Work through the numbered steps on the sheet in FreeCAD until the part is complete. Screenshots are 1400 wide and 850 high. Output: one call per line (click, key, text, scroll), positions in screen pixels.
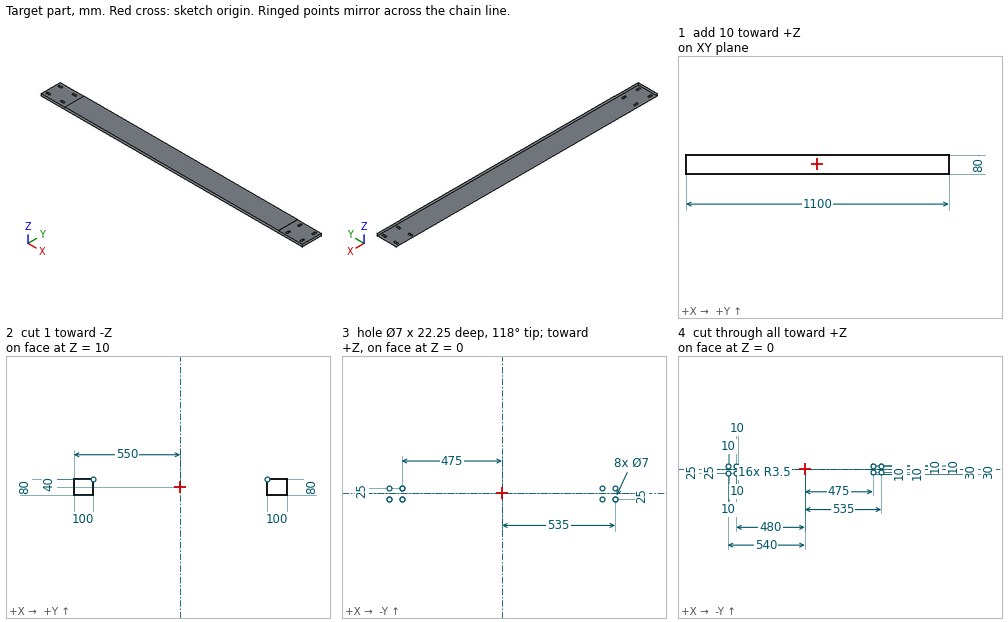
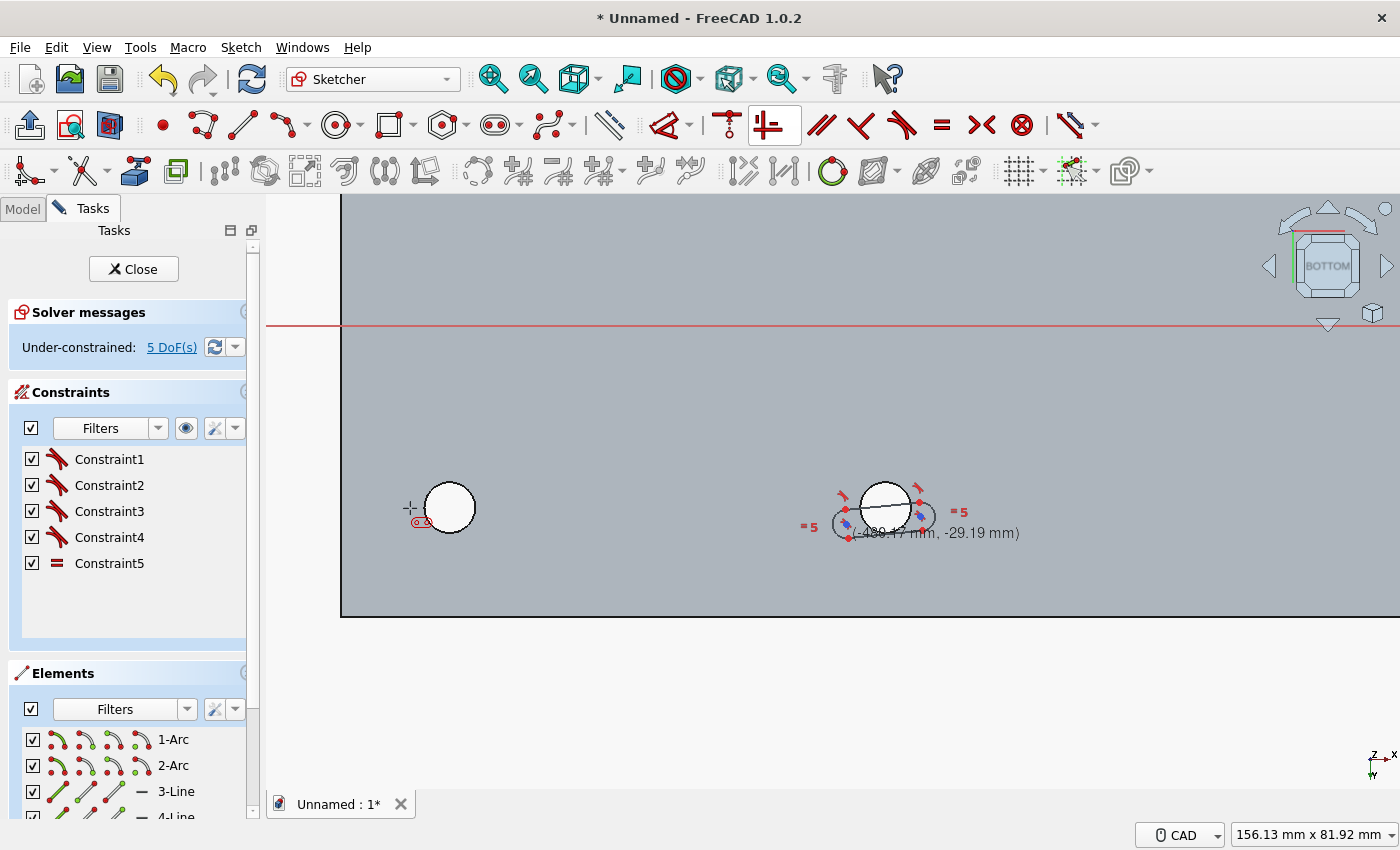
scroll(410, 508, down, 12)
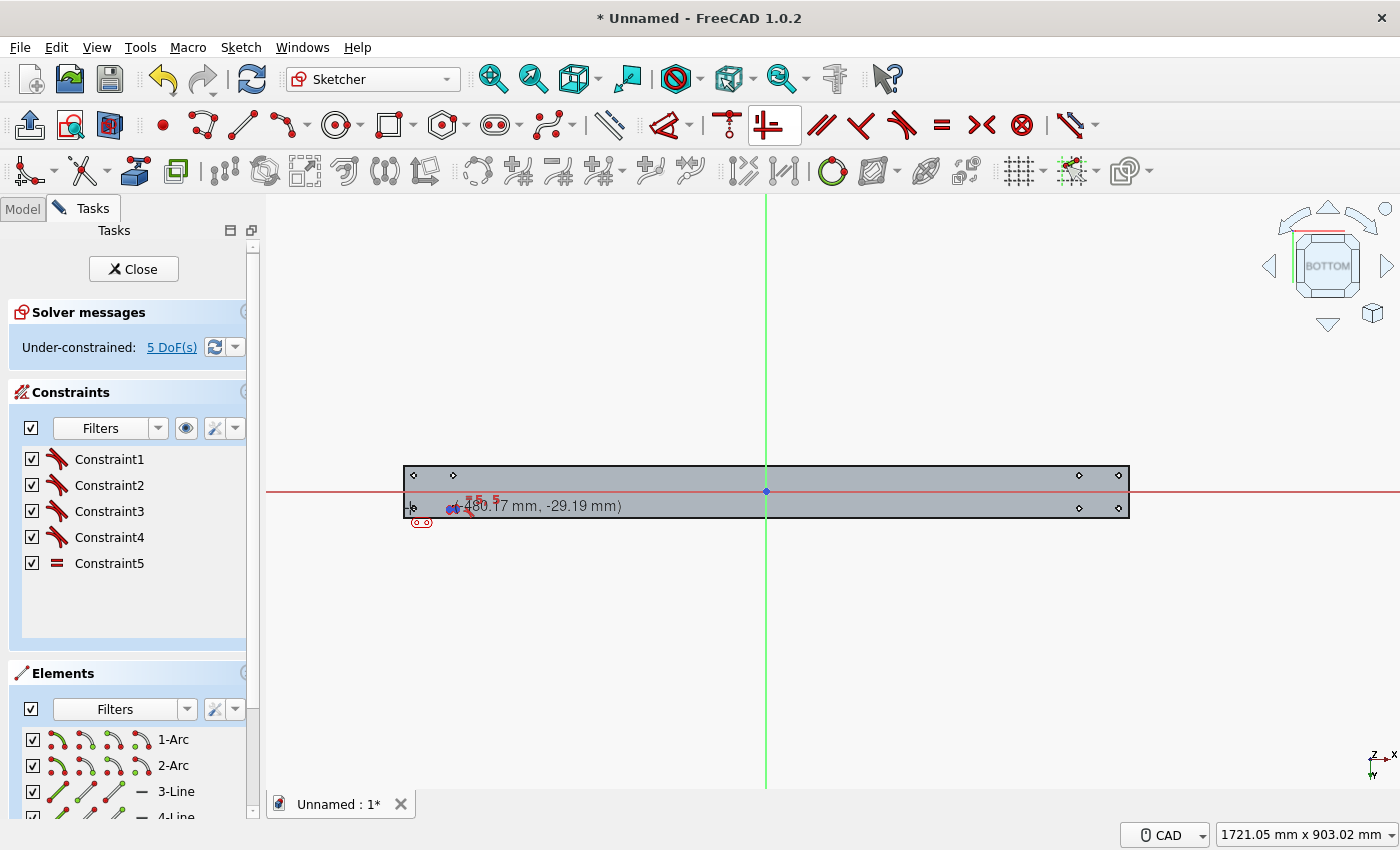
click(410, 508)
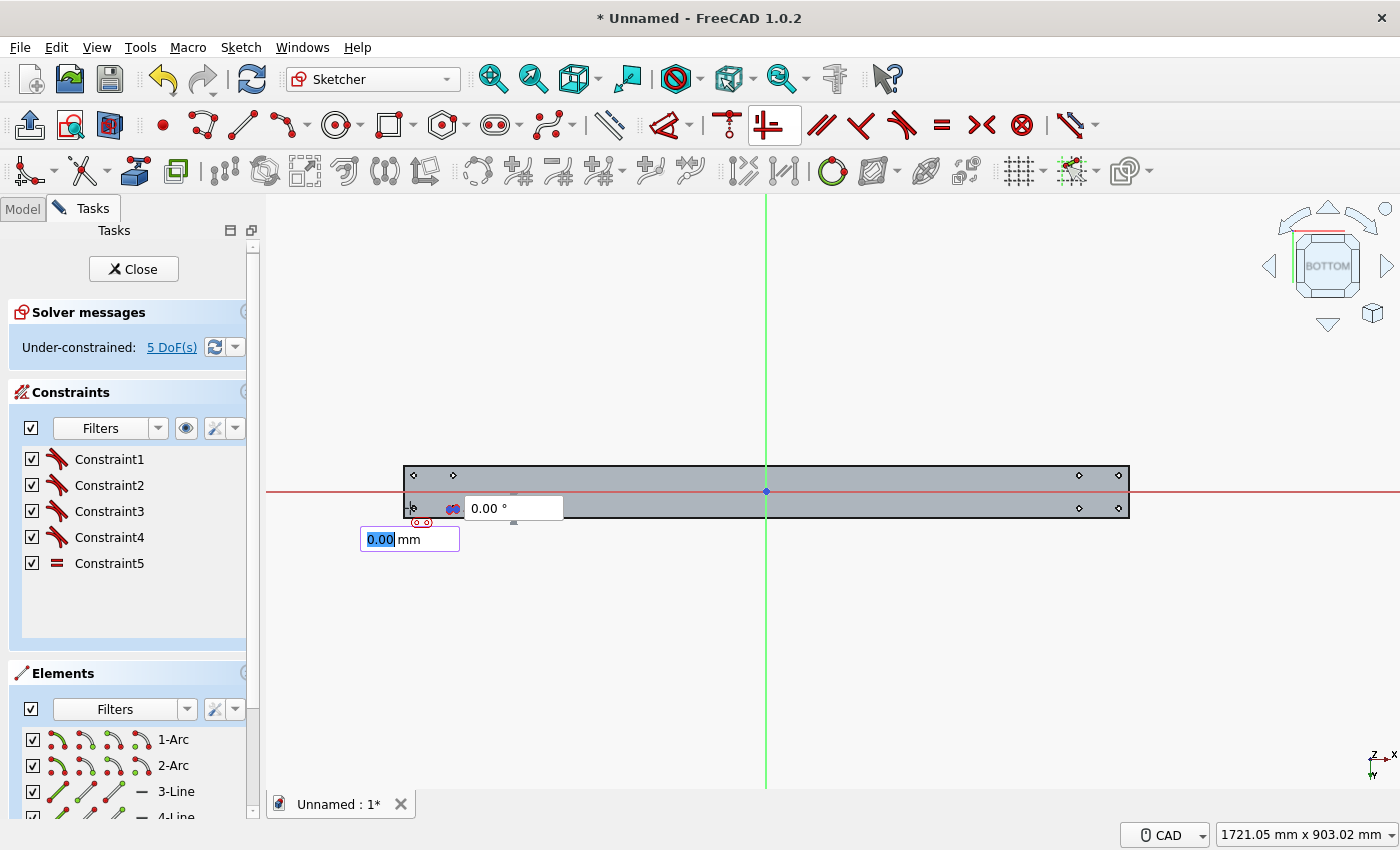
scroll(417, 508, up, 5)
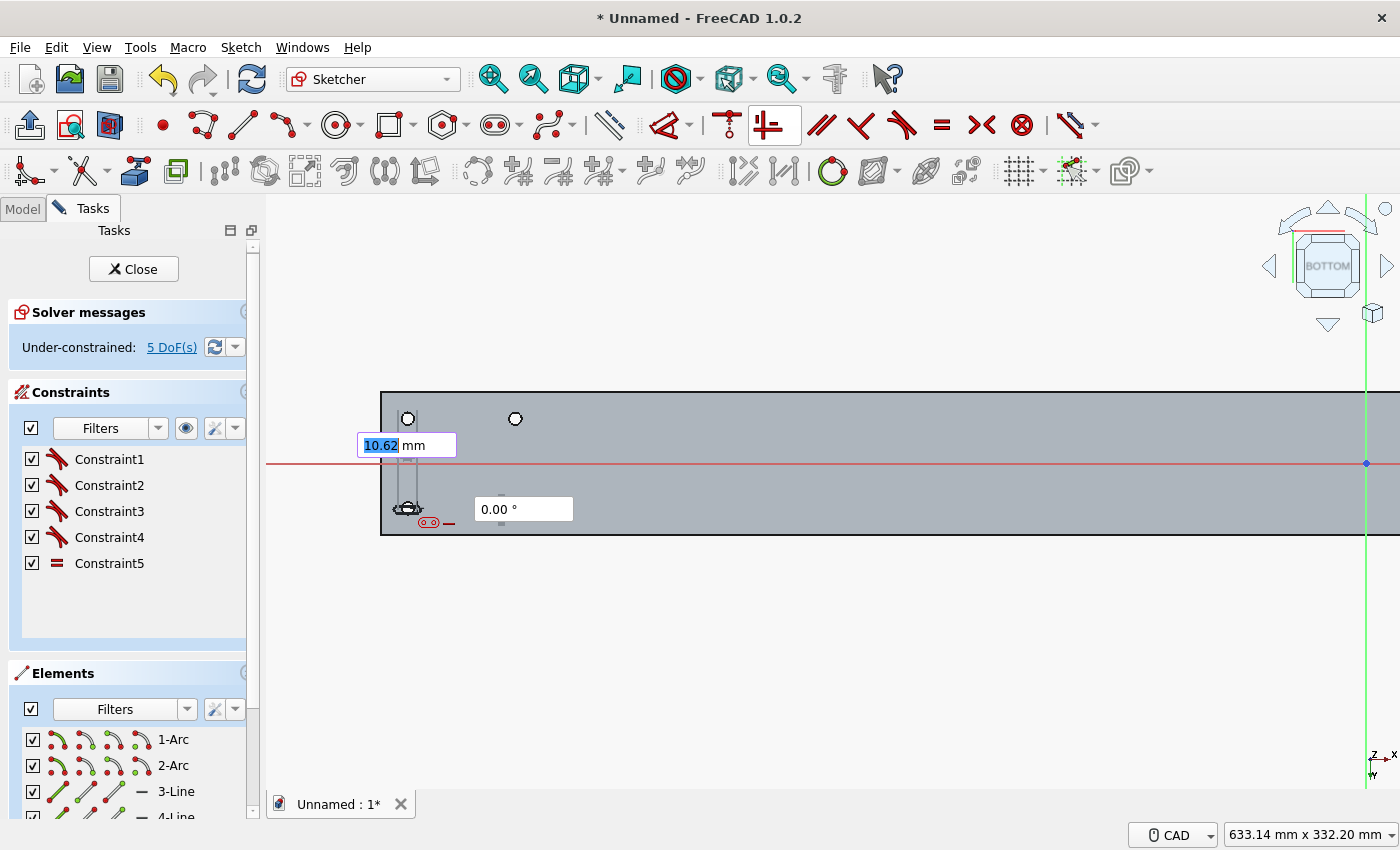
click(417, 507)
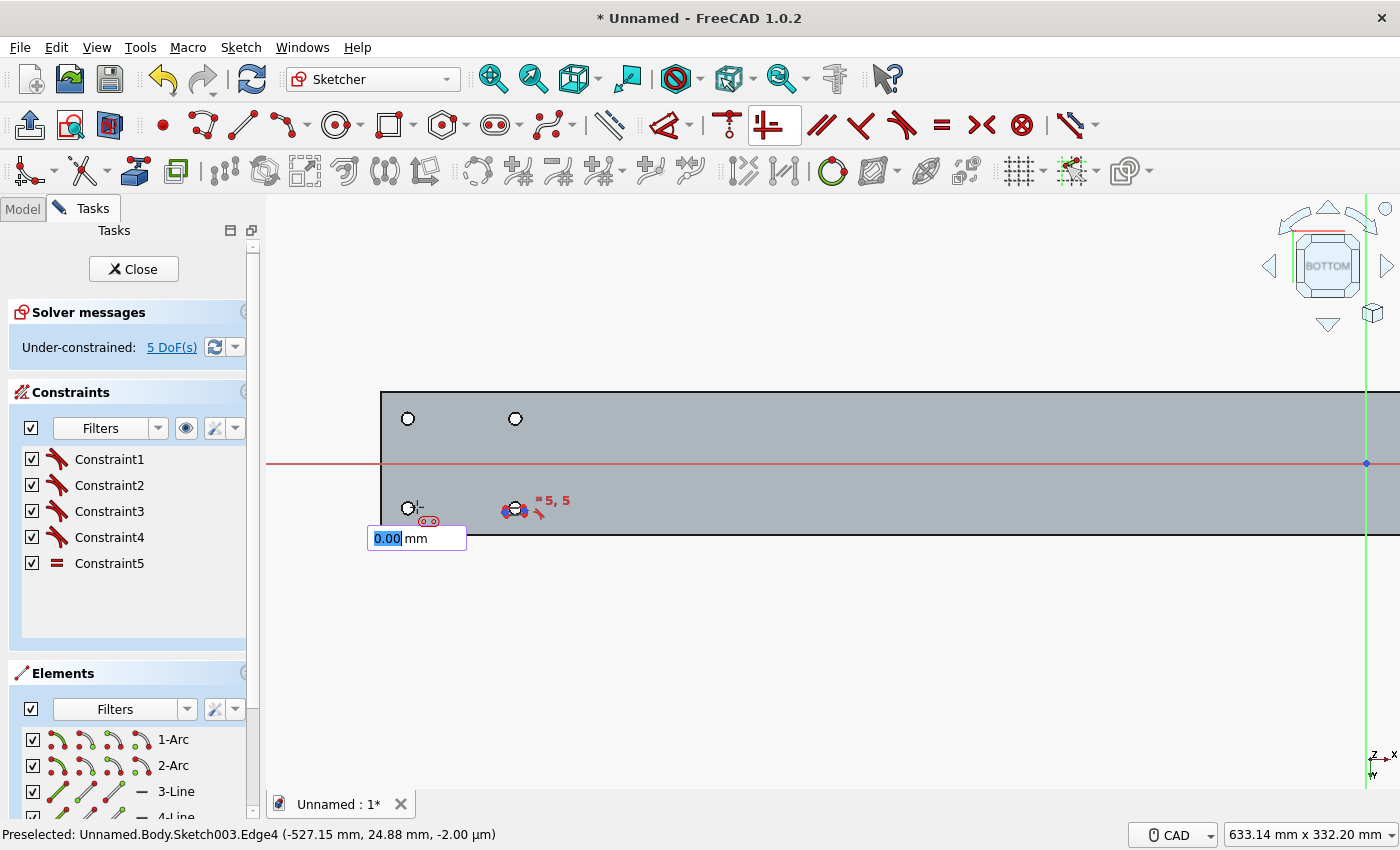
scroll(408, 515, up, 5)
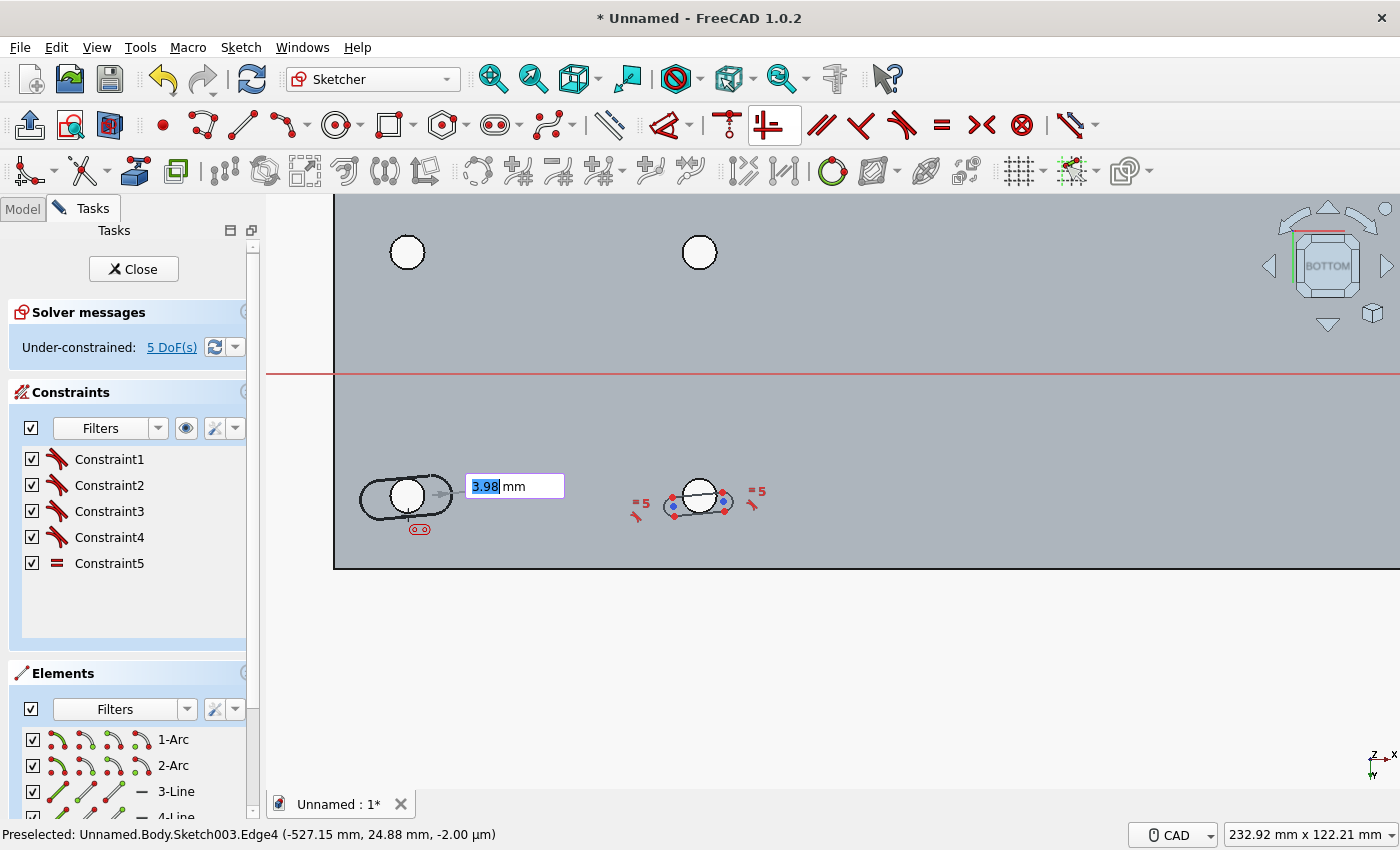
click(407, 513)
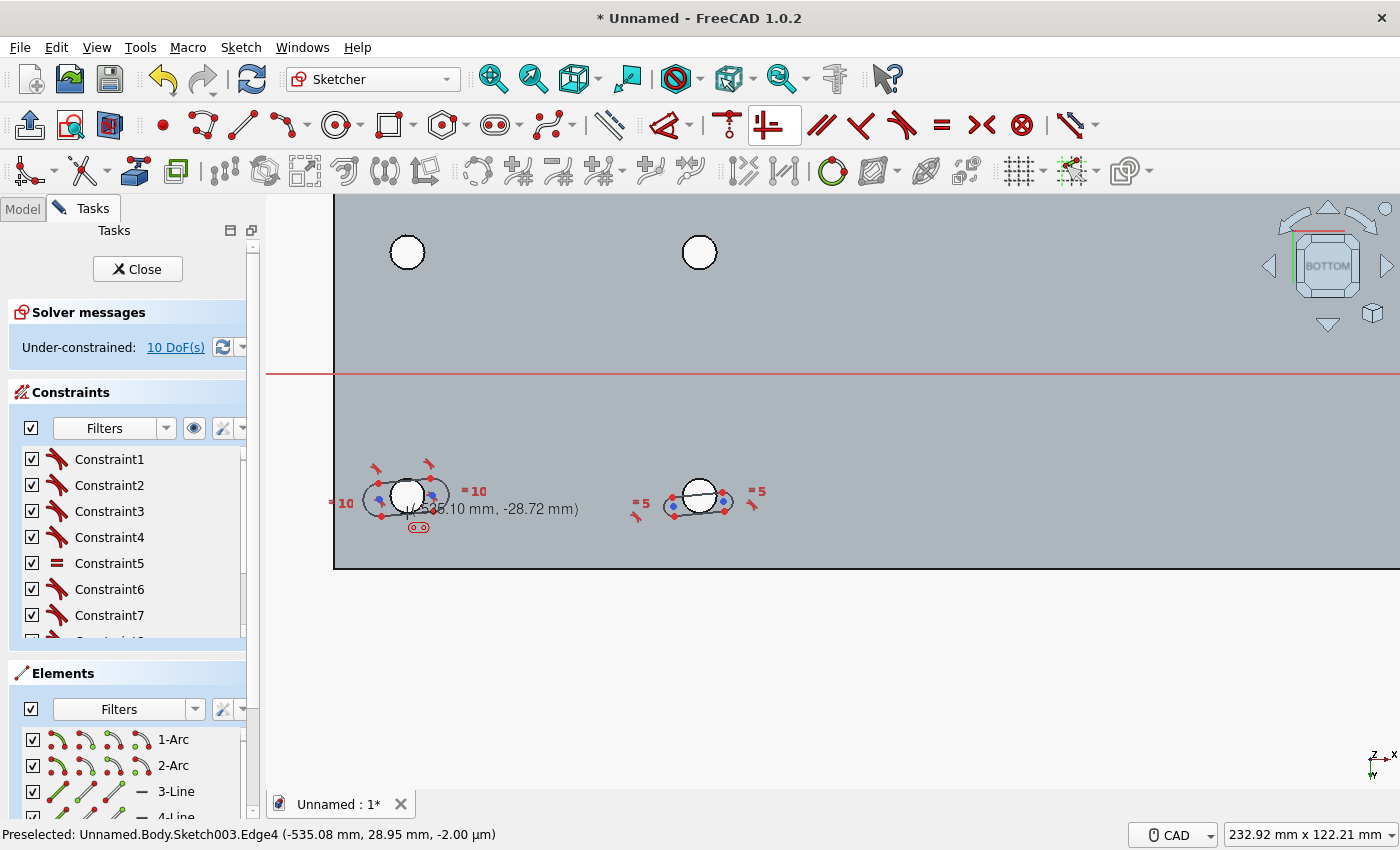
scroll(383, 252, up, 2)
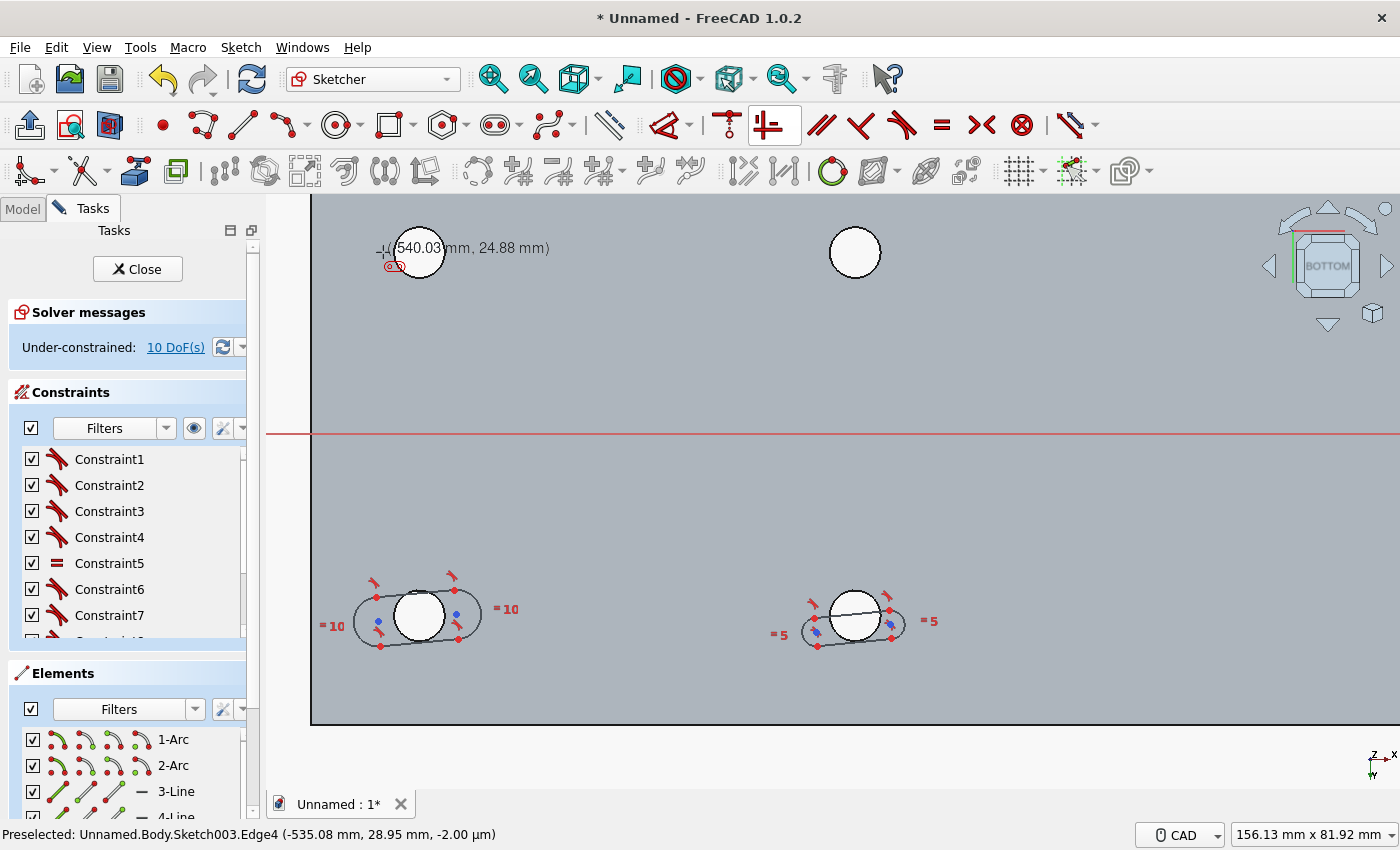
scroll(413, 497, down, 12)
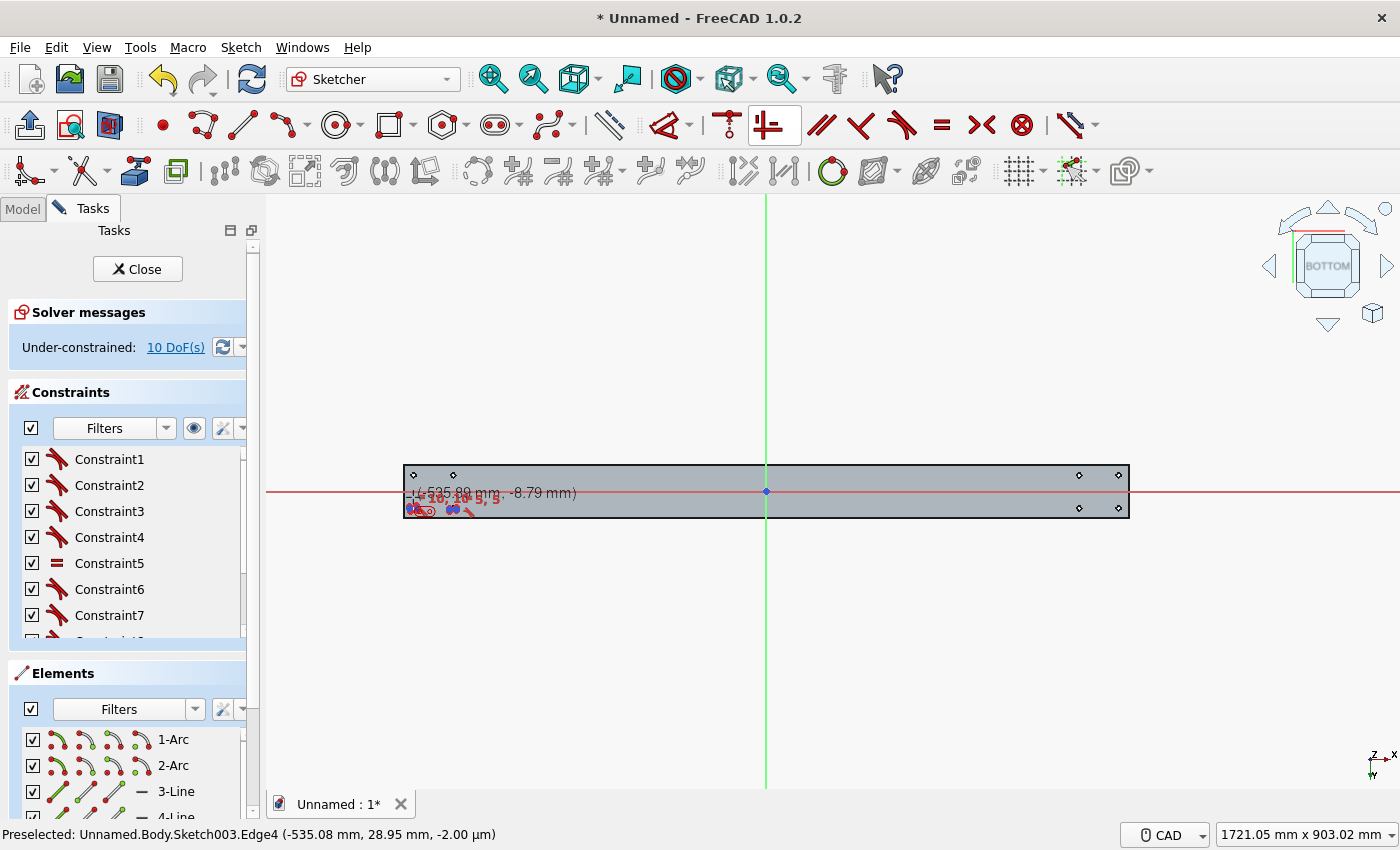
click(410, 475)